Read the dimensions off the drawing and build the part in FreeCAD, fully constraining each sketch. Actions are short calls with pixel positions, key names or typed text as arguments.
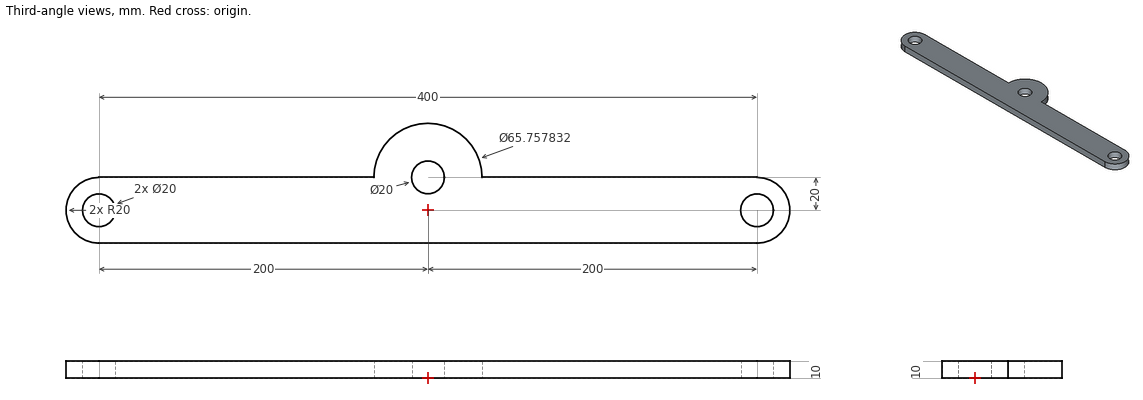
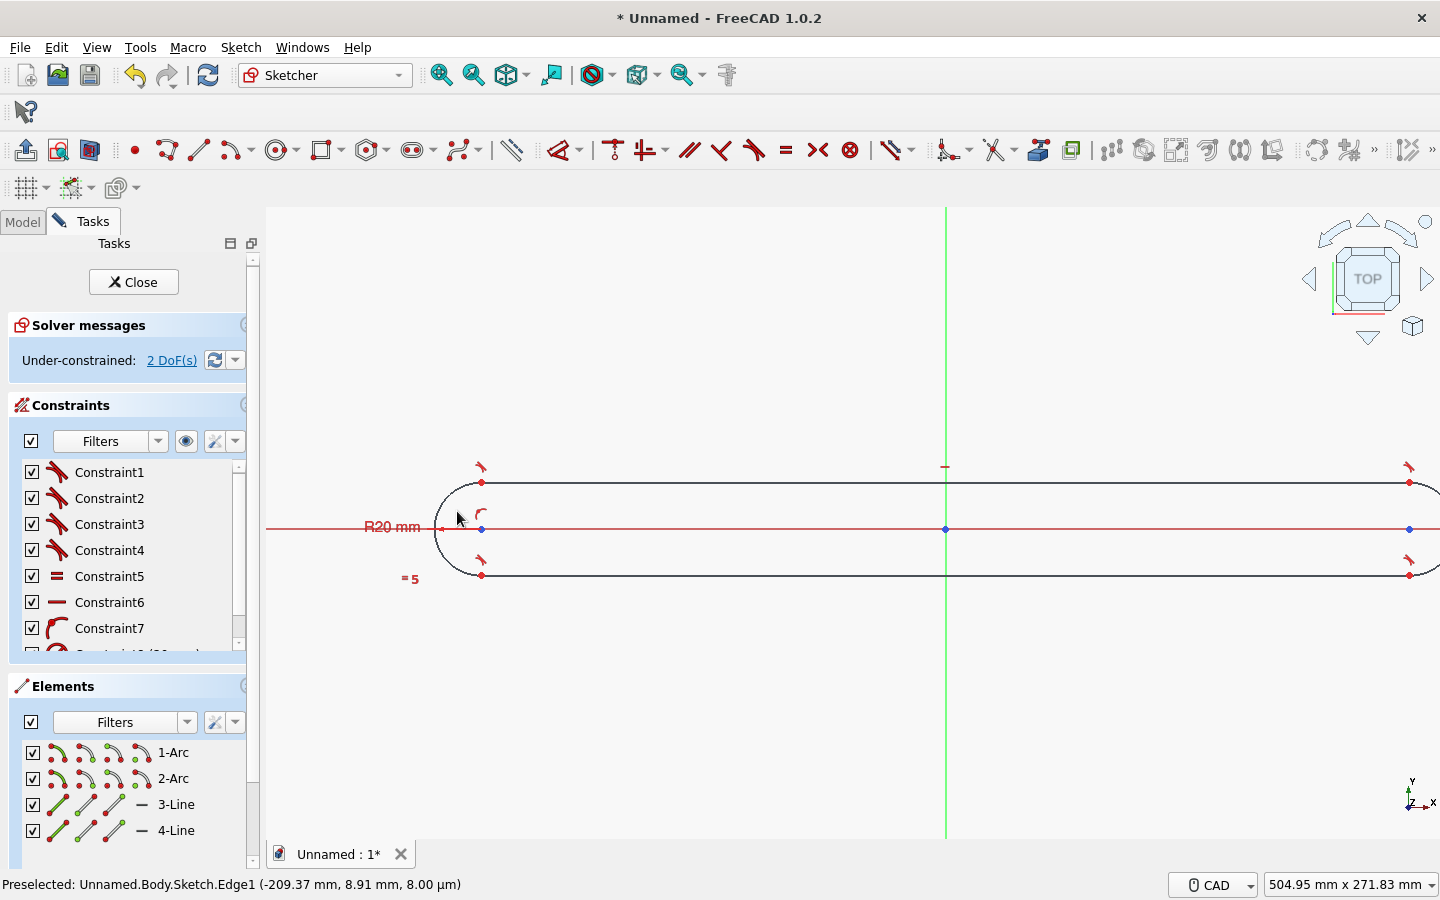
click(760, 483)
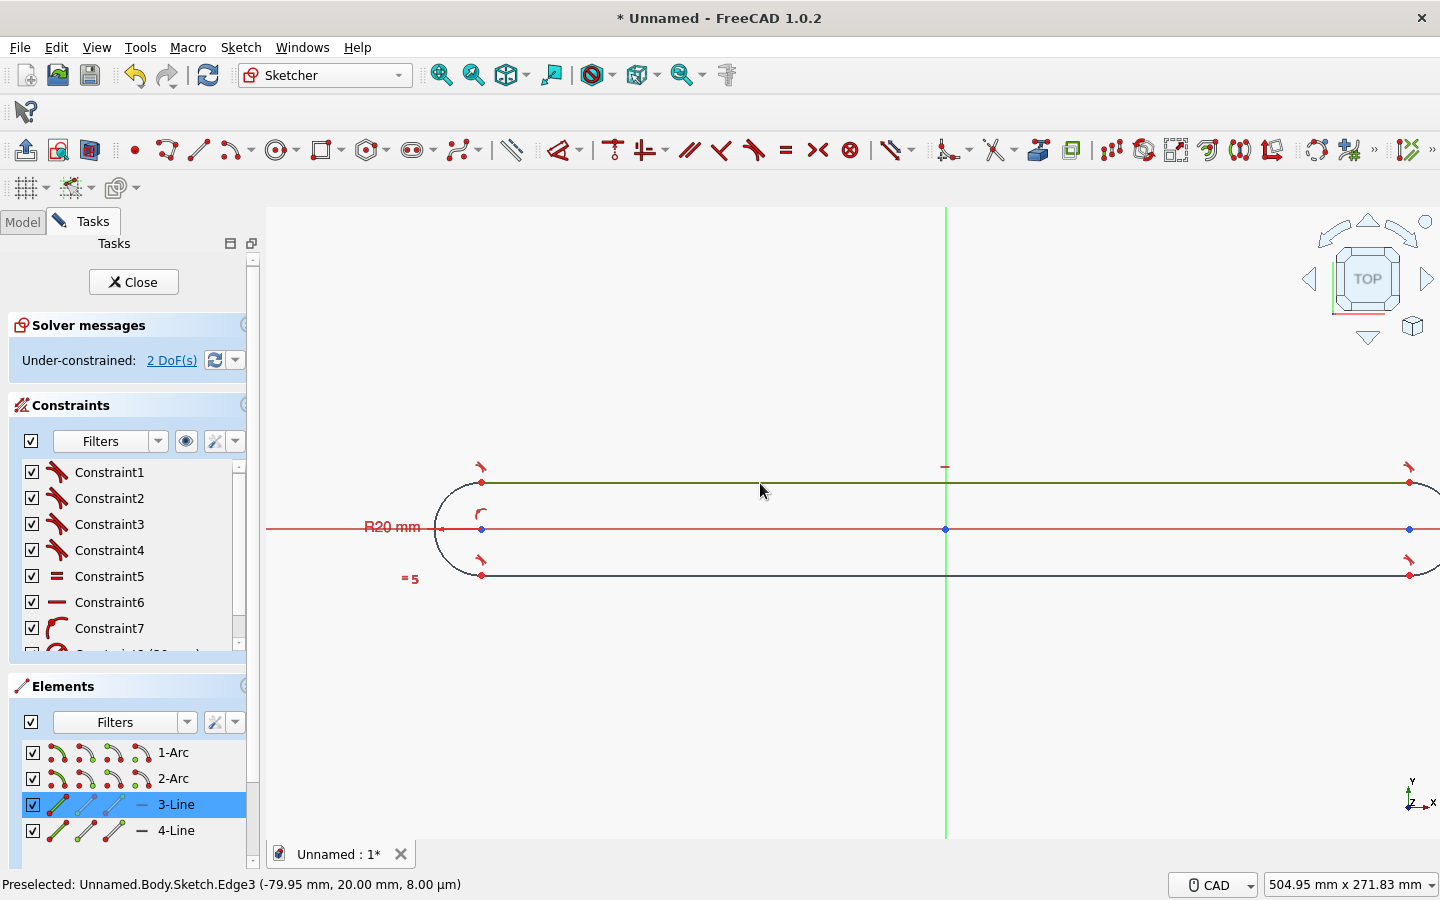
click(582, 150)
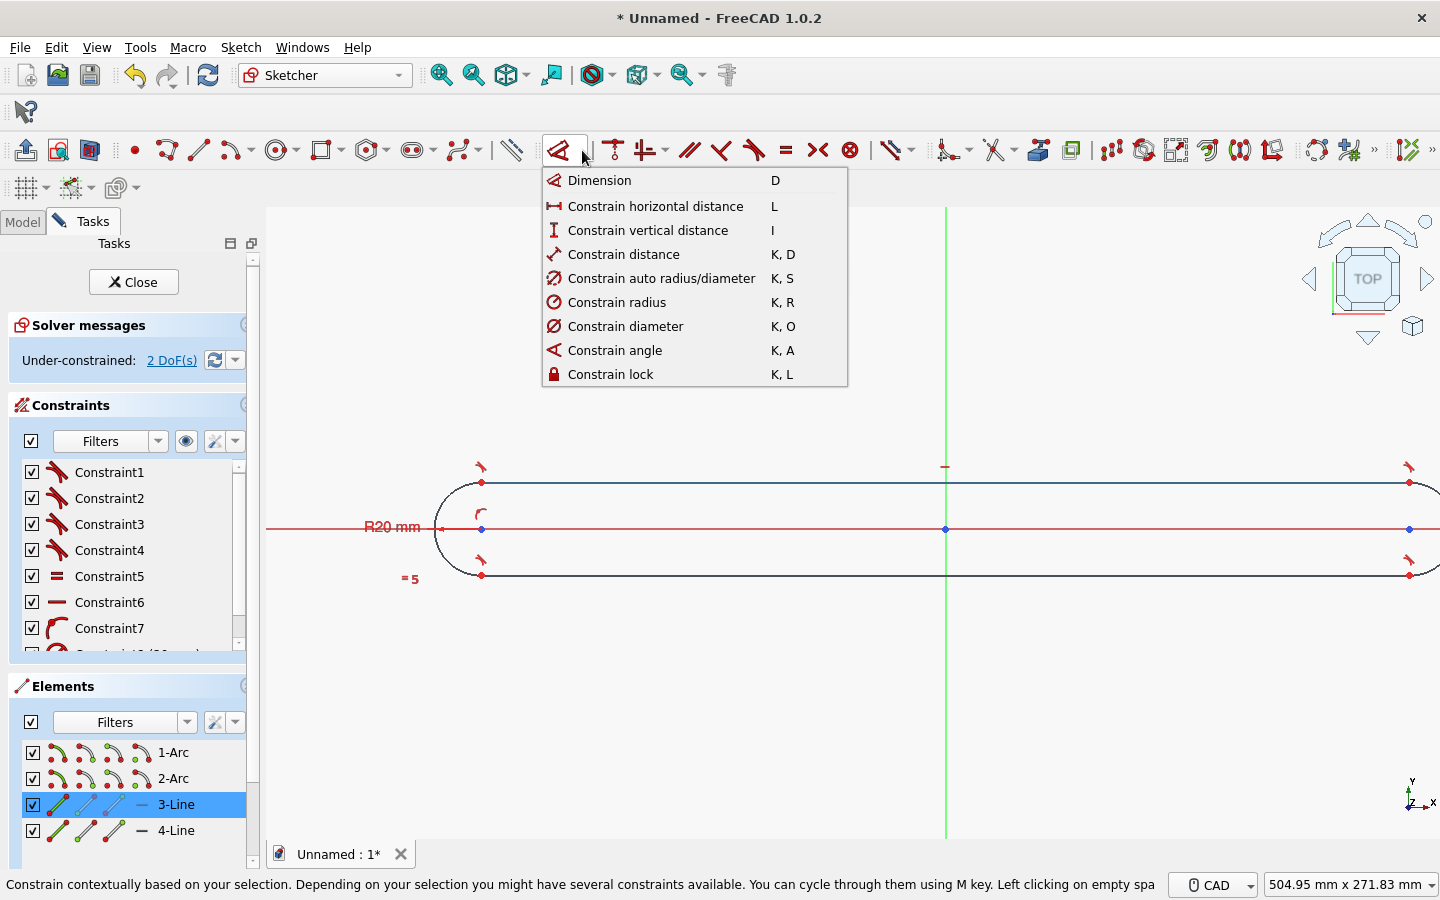
click(695, 206)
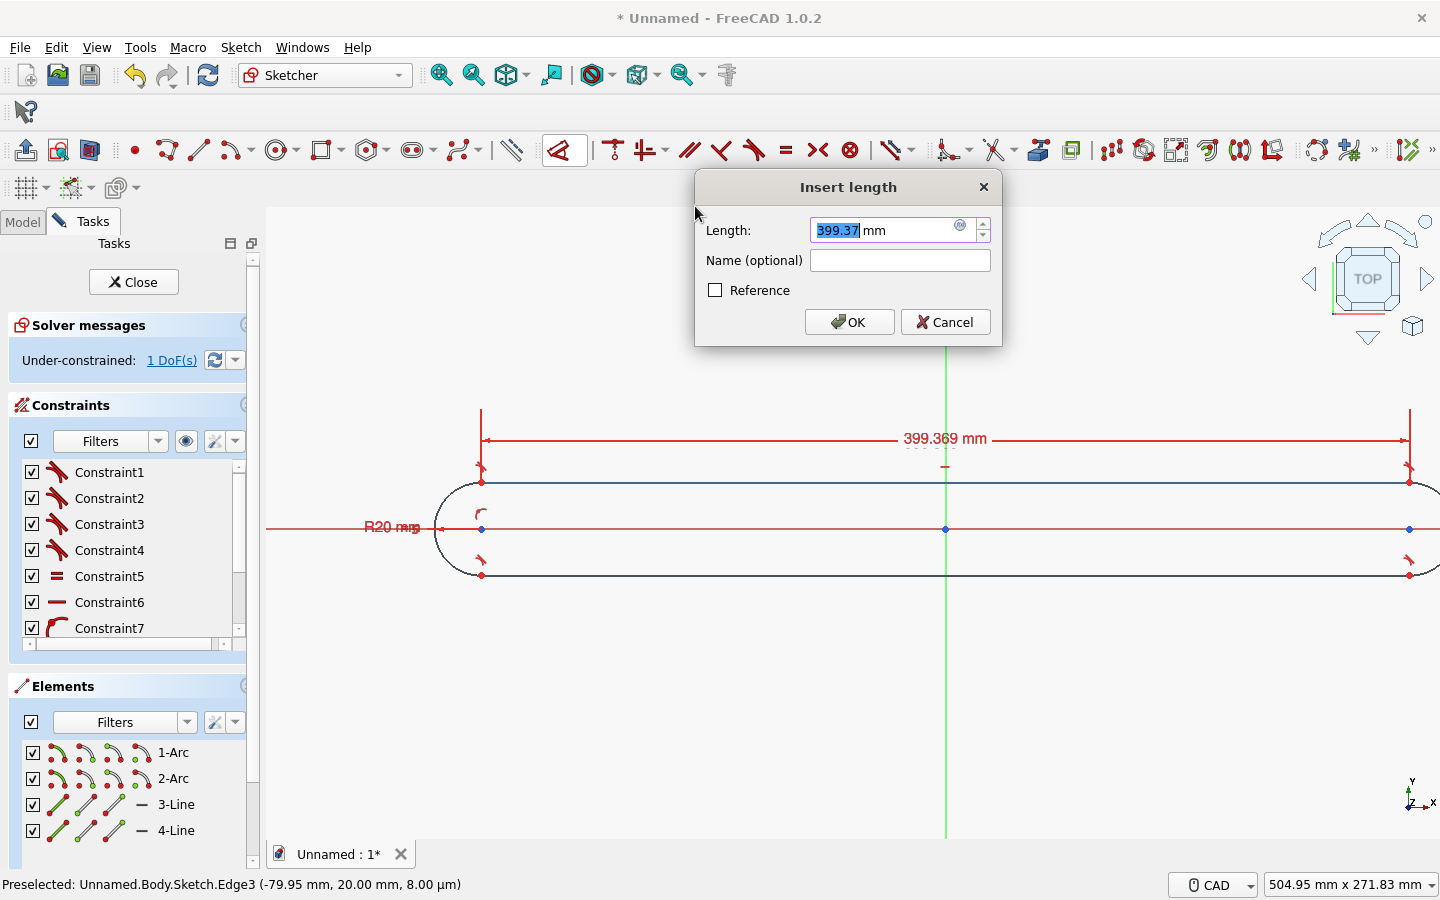
text(400)
key(Return)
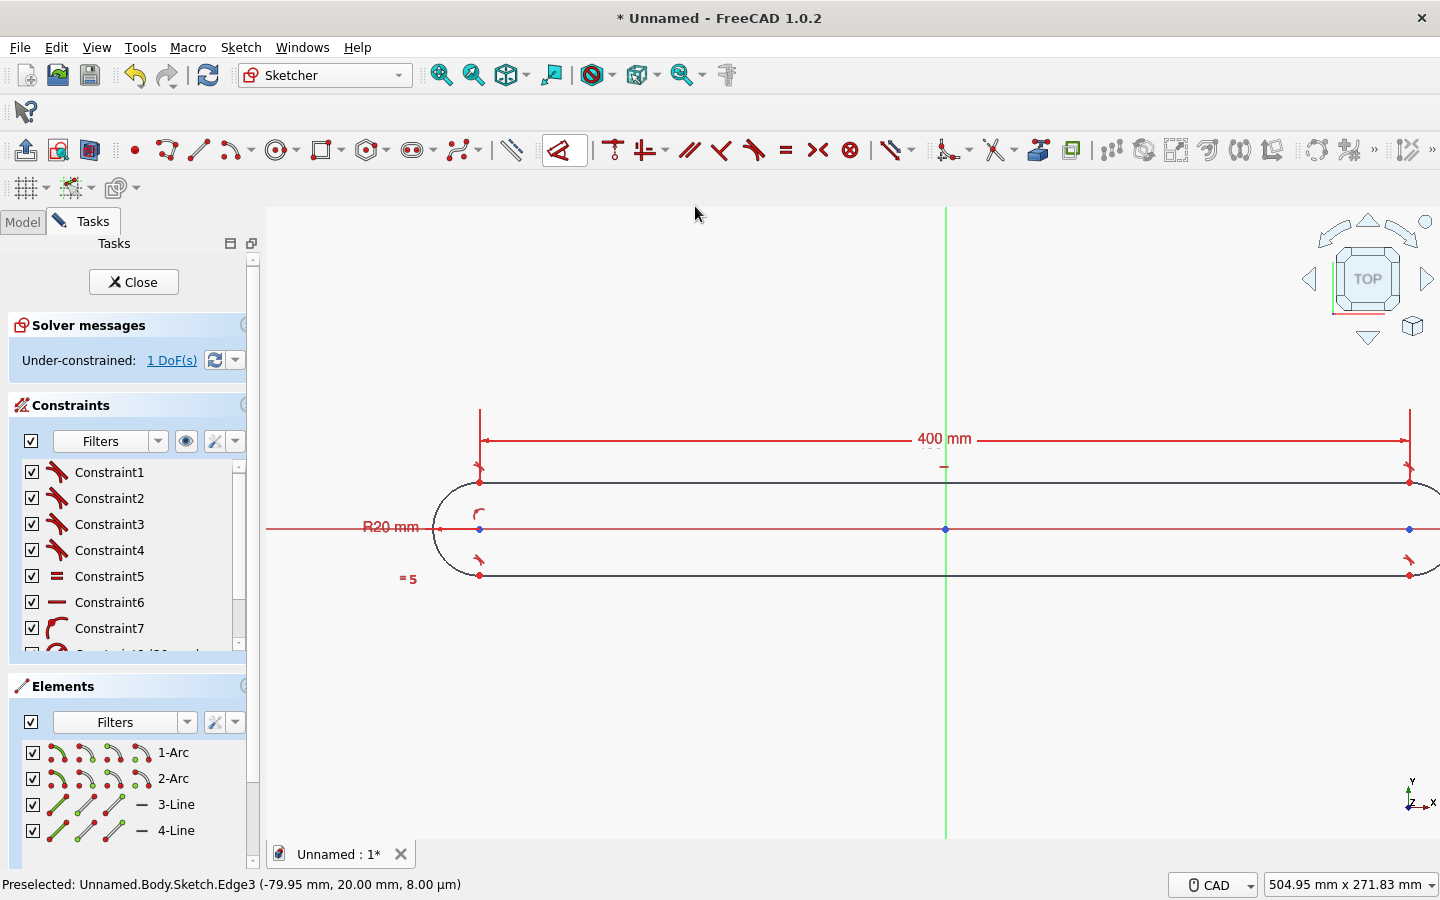
click(480, 483)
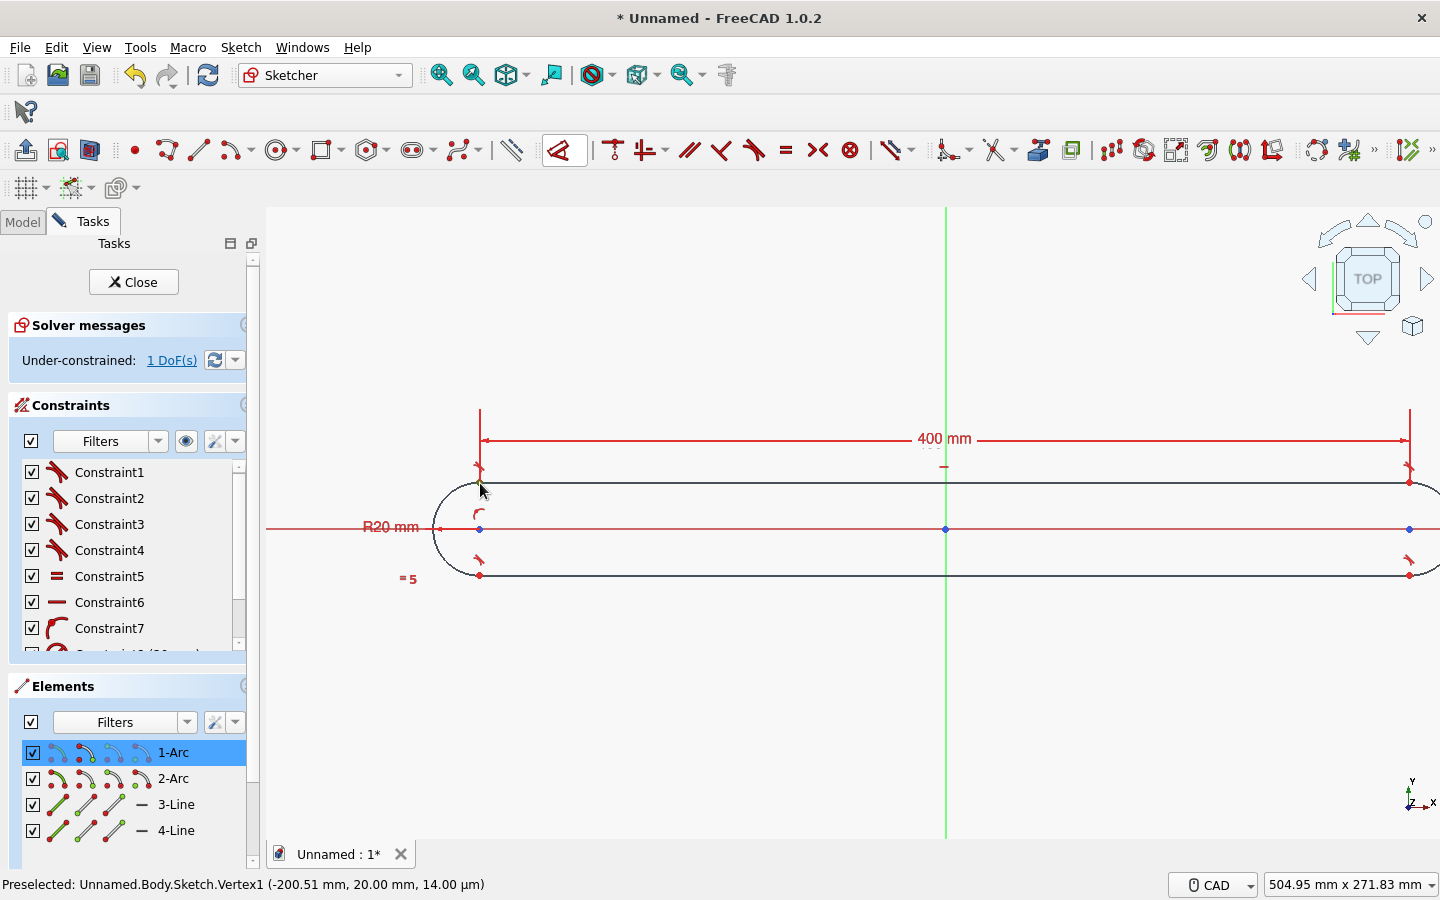
click(582, 150)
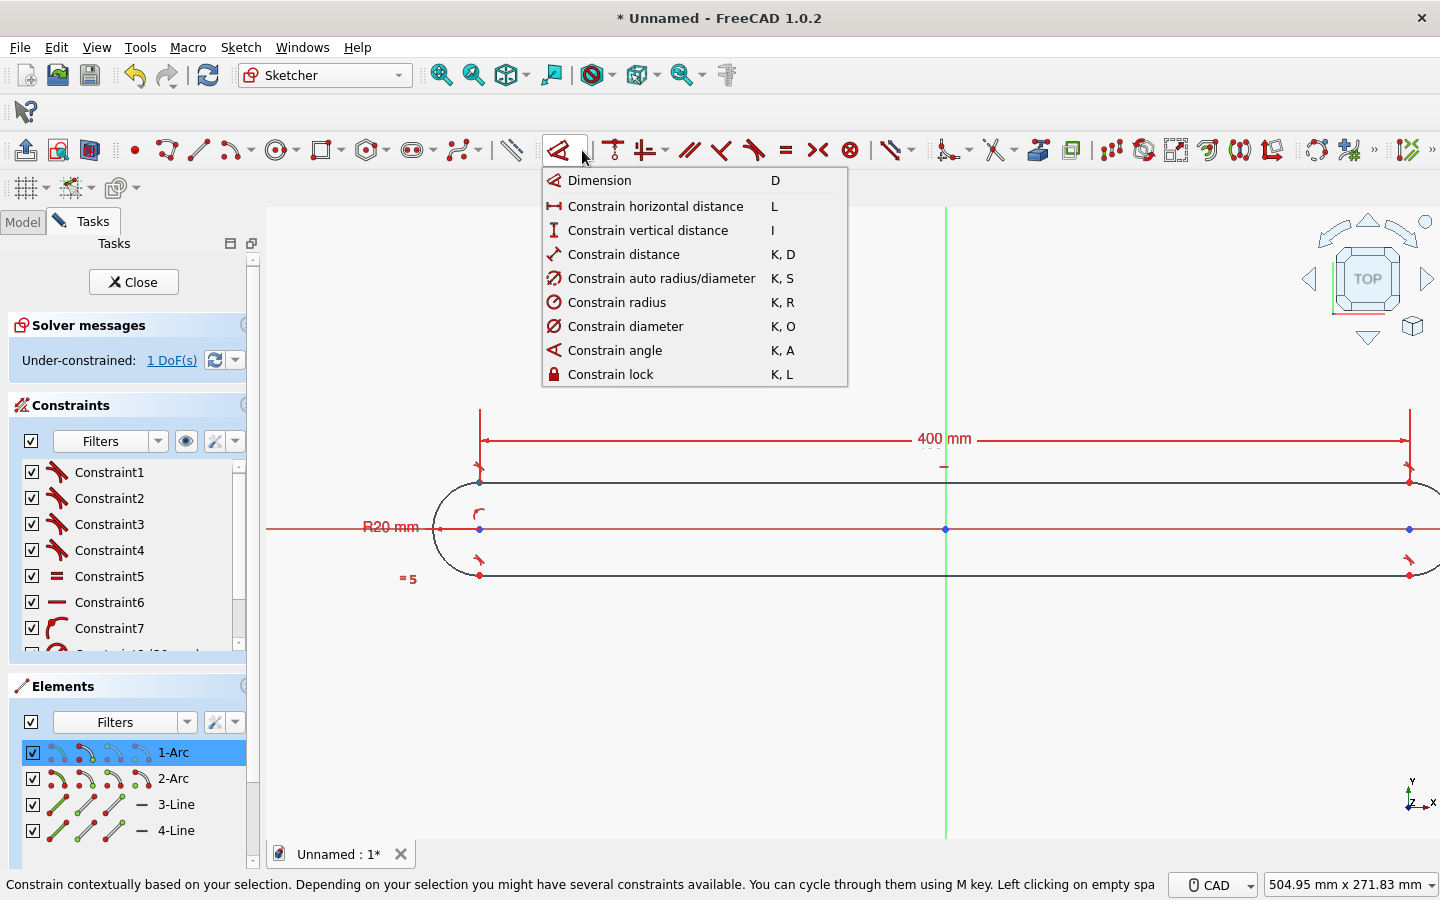
click(695, 206)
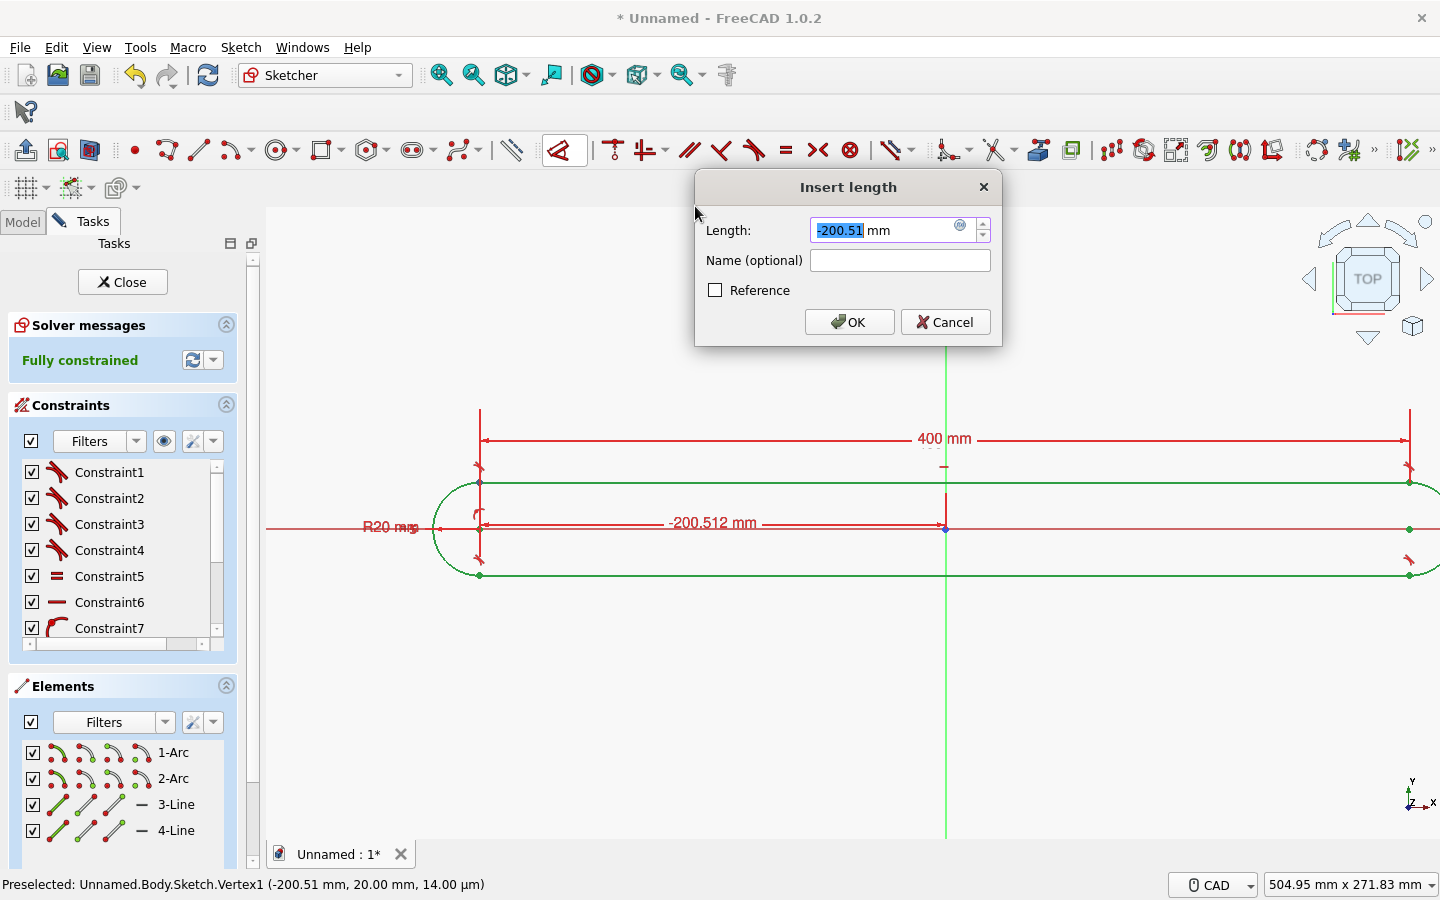
text(-200)
key(Return)